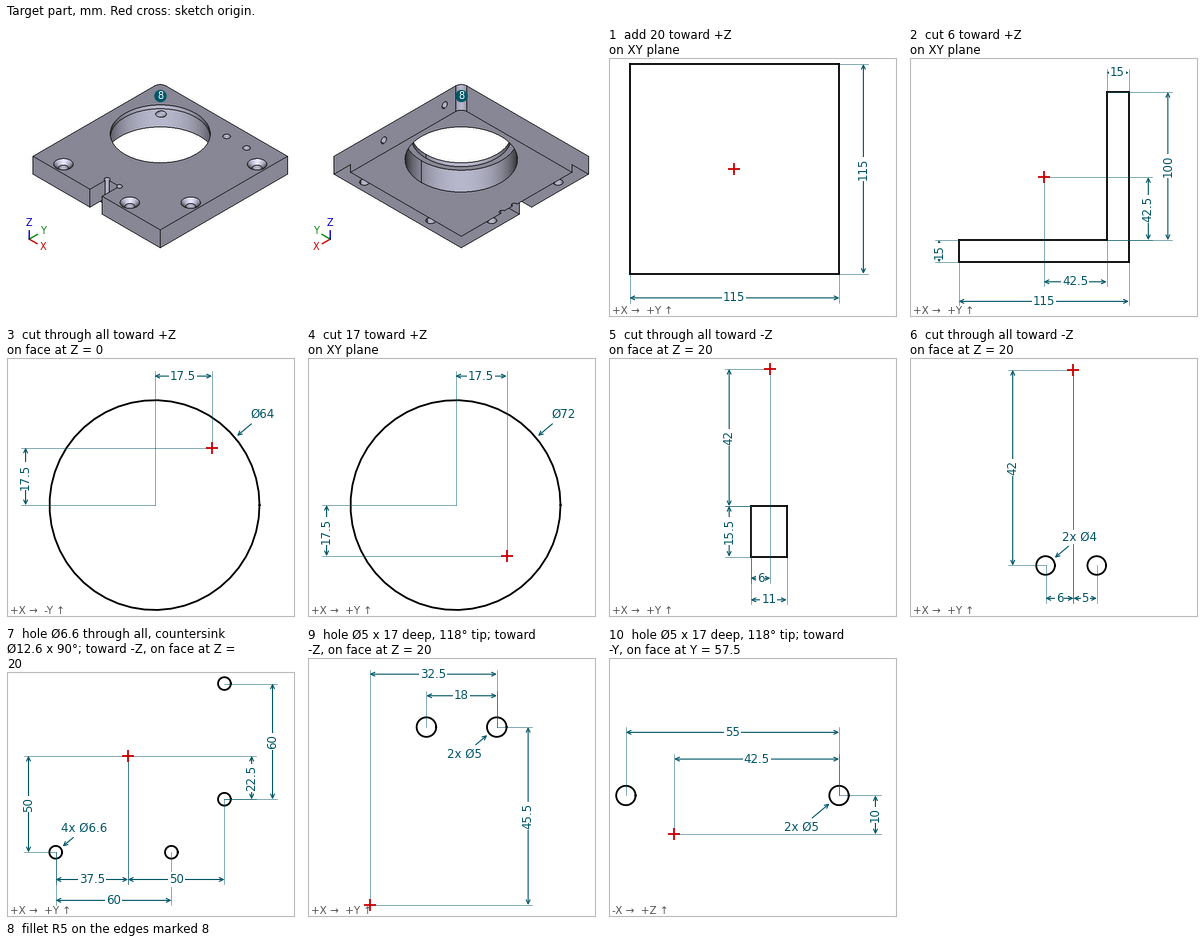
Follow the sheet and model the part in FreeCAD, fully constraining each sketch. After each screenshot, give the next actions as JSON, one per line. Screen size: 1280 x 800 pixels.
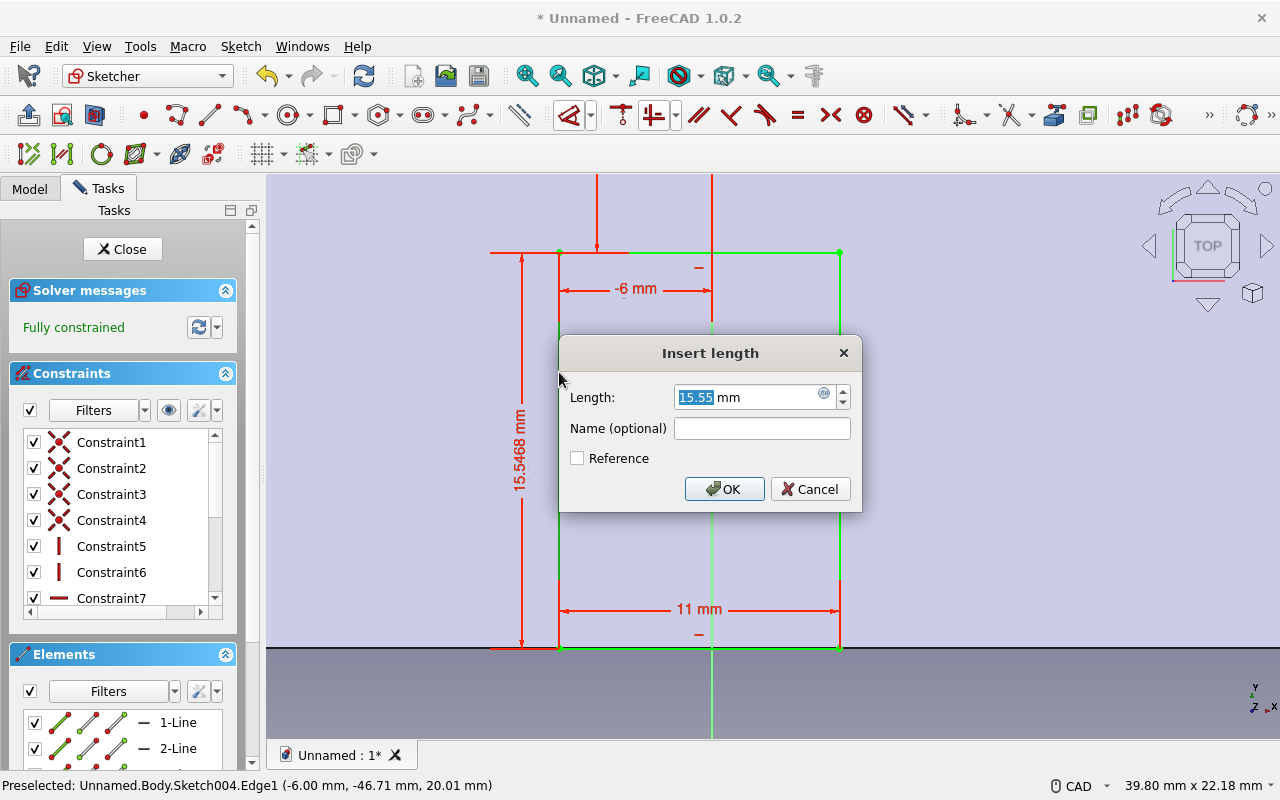
{"action": "type", "text": "15.5"}
{"action": "key", "text": "Return"}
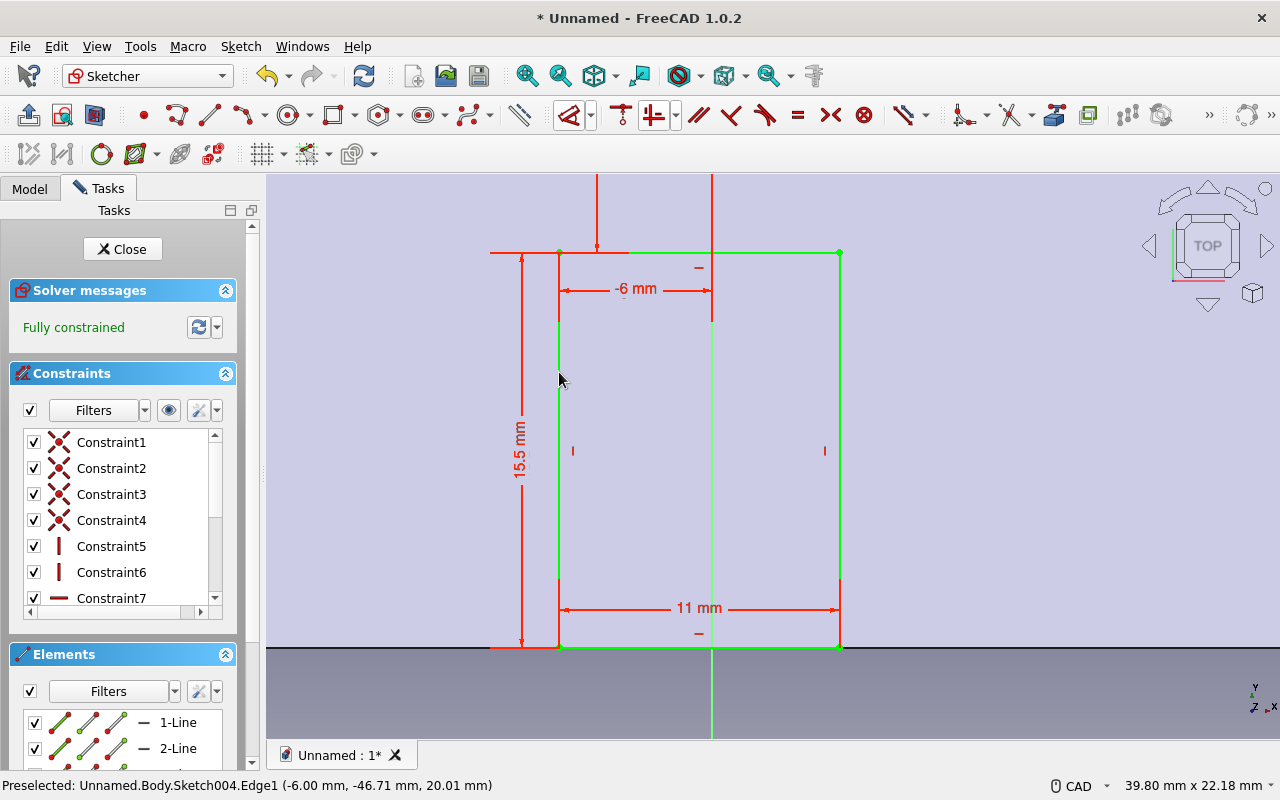
{"action": "left_click", "coordinate": [123, 249]}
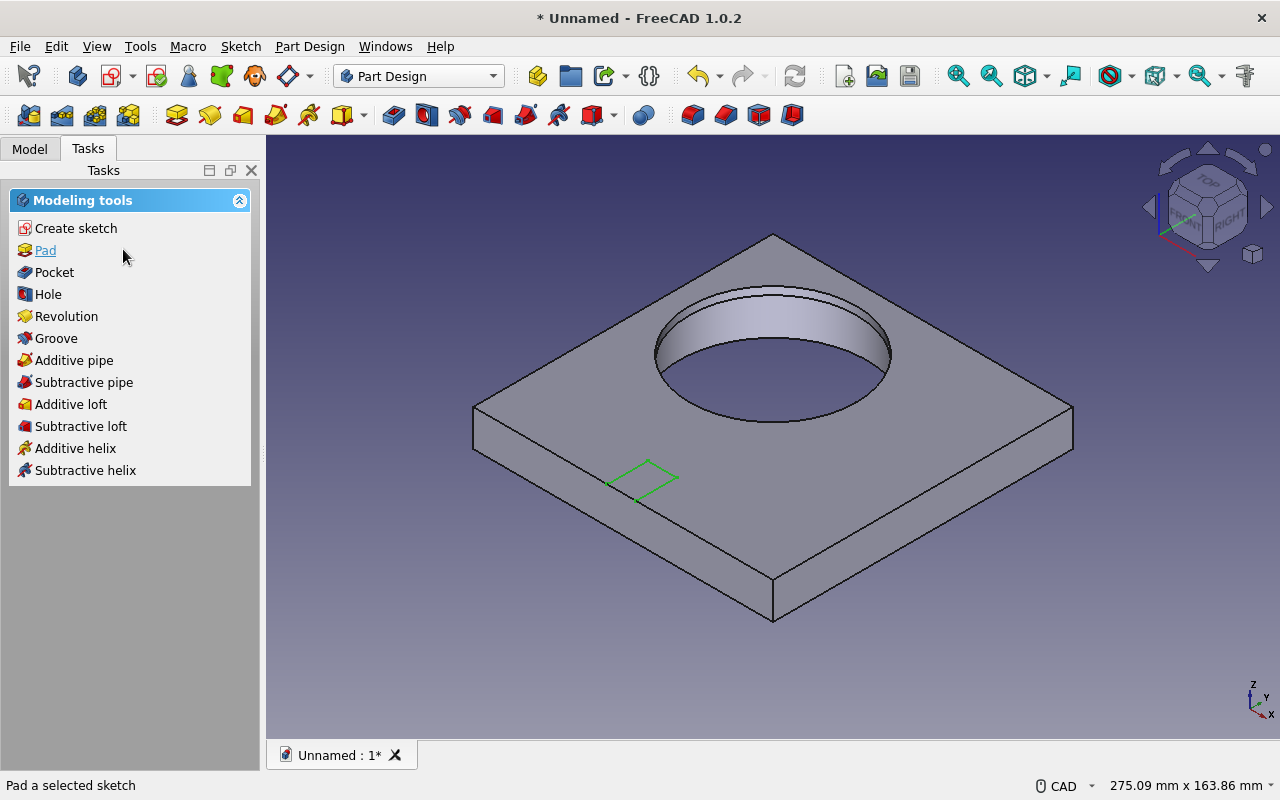
{"action": "left_click", "coordinate": [394, 116]}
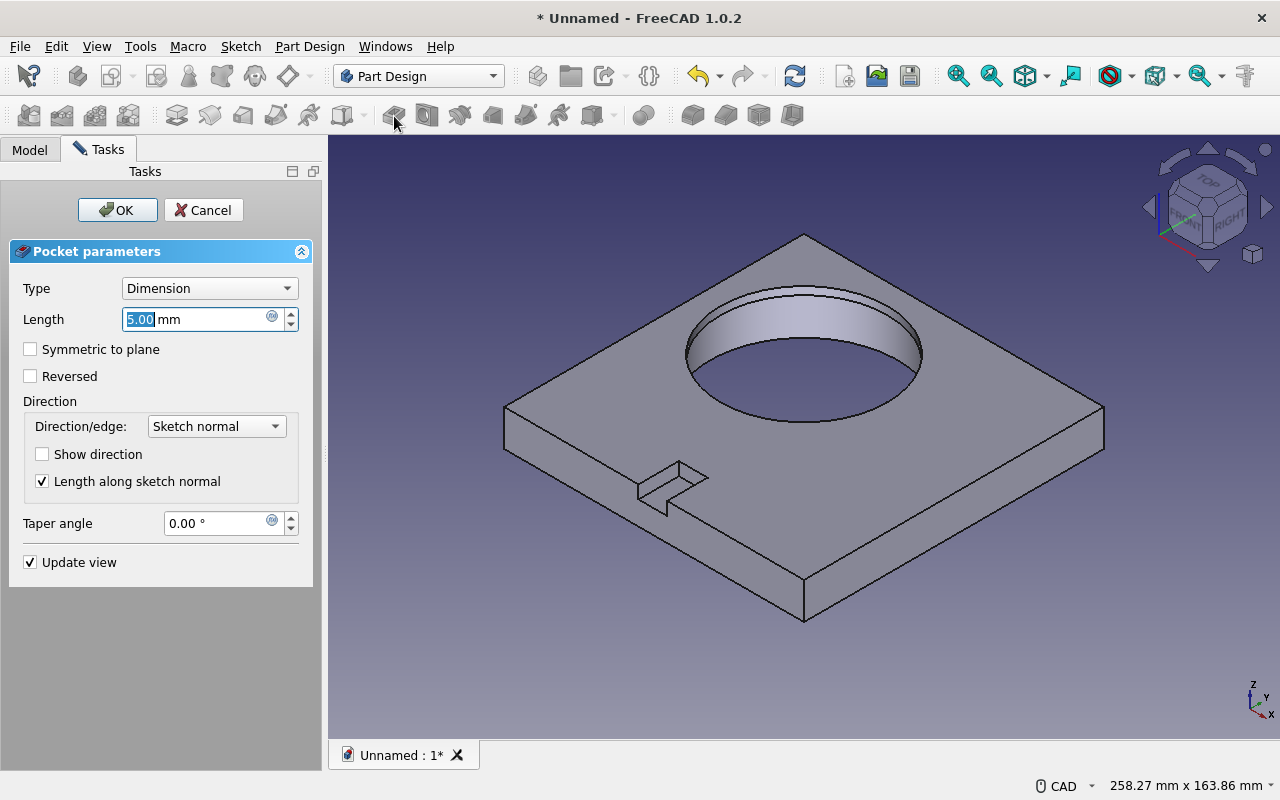
{"action": "left_click", "coordinate": [210, 288]}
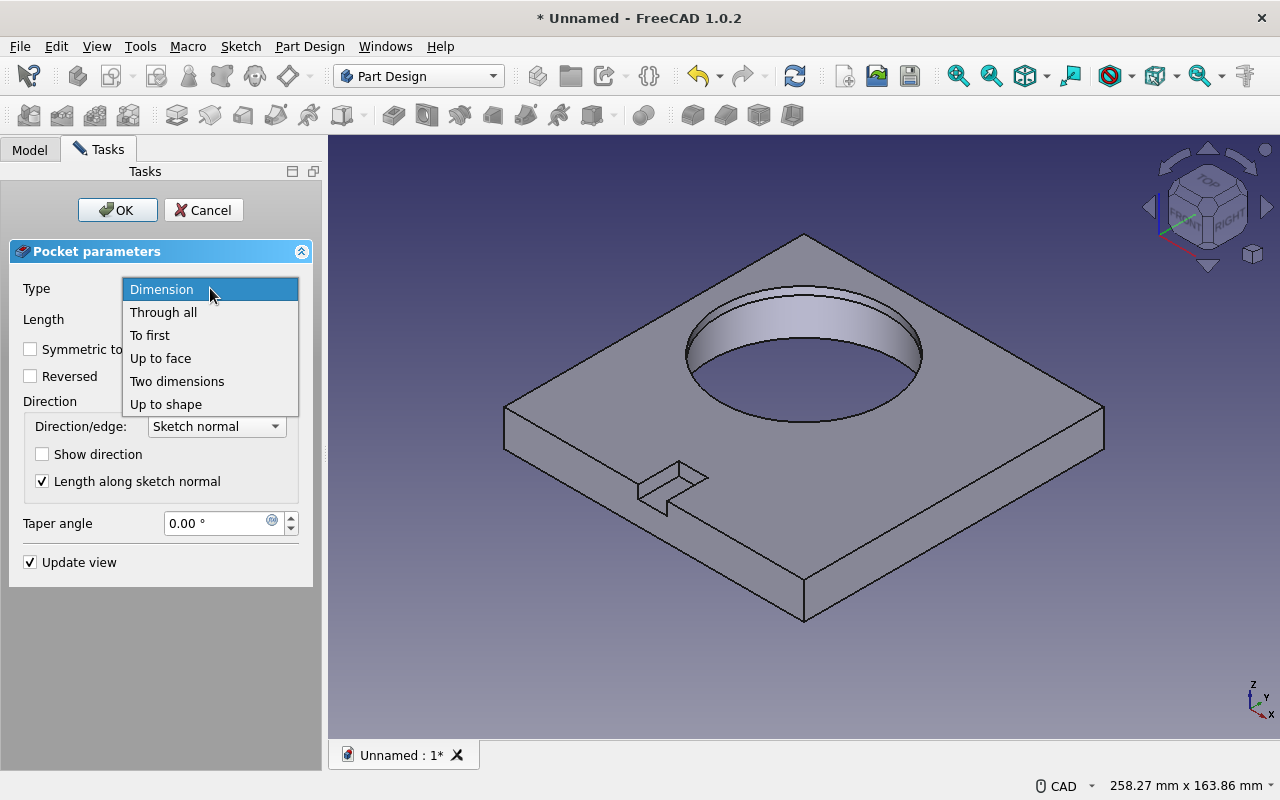
{"action": "left_click", "coordinate": [208, 312]}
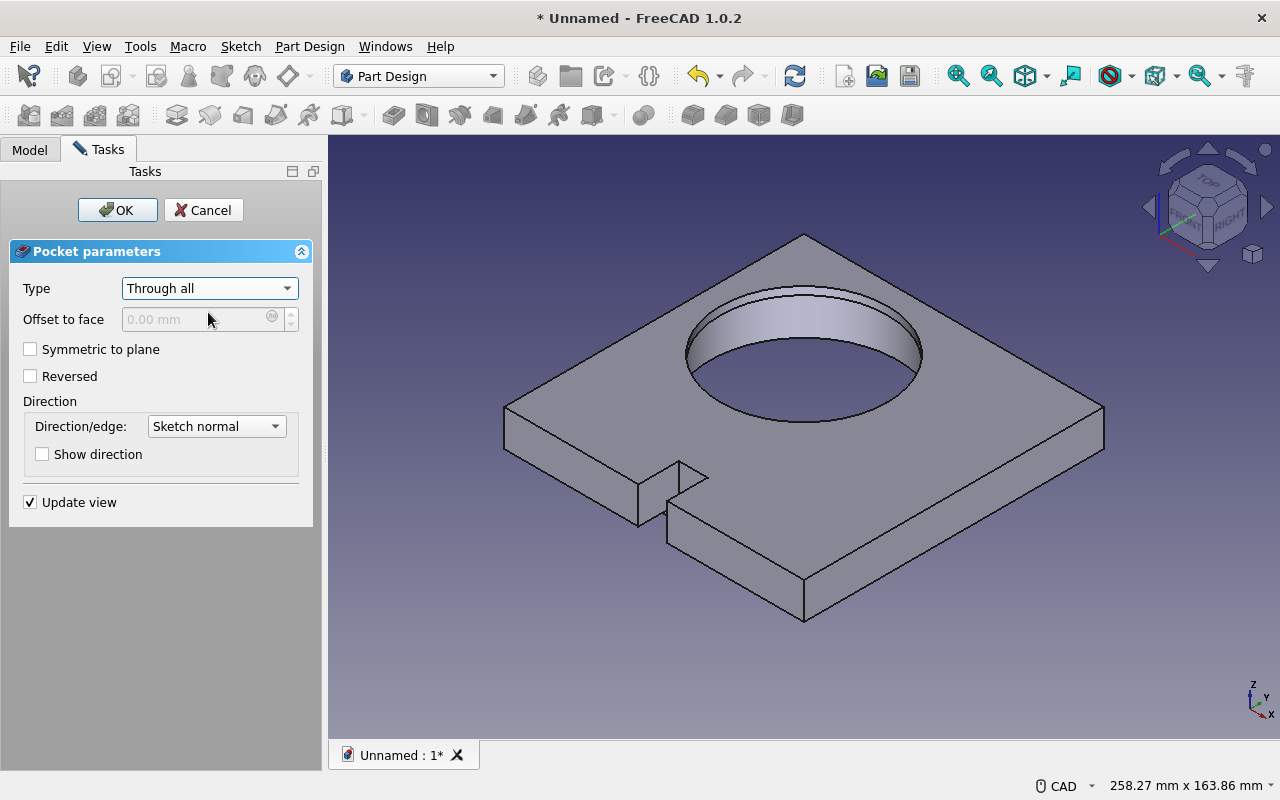
{"action": "left_click", "coordinate": [118, 210]}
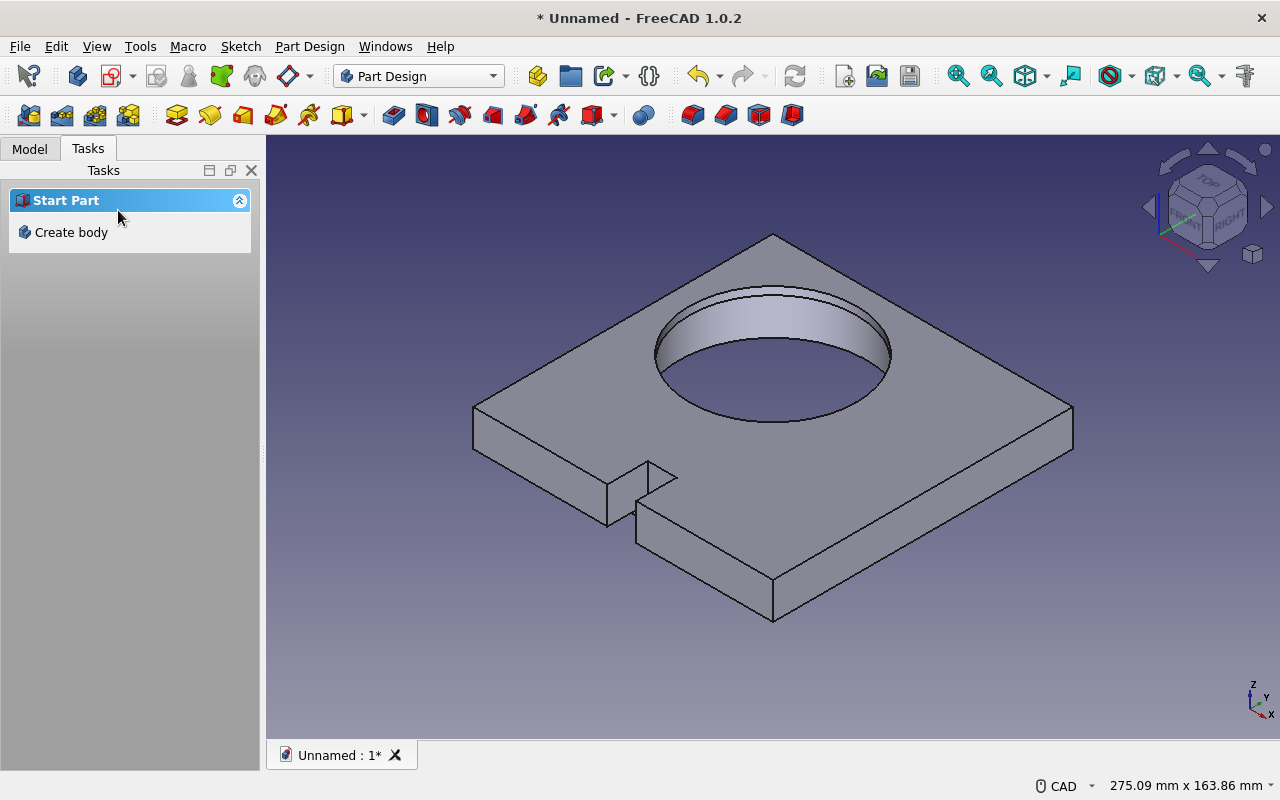
{"action": "left_click", "coordinate": [816, 480]}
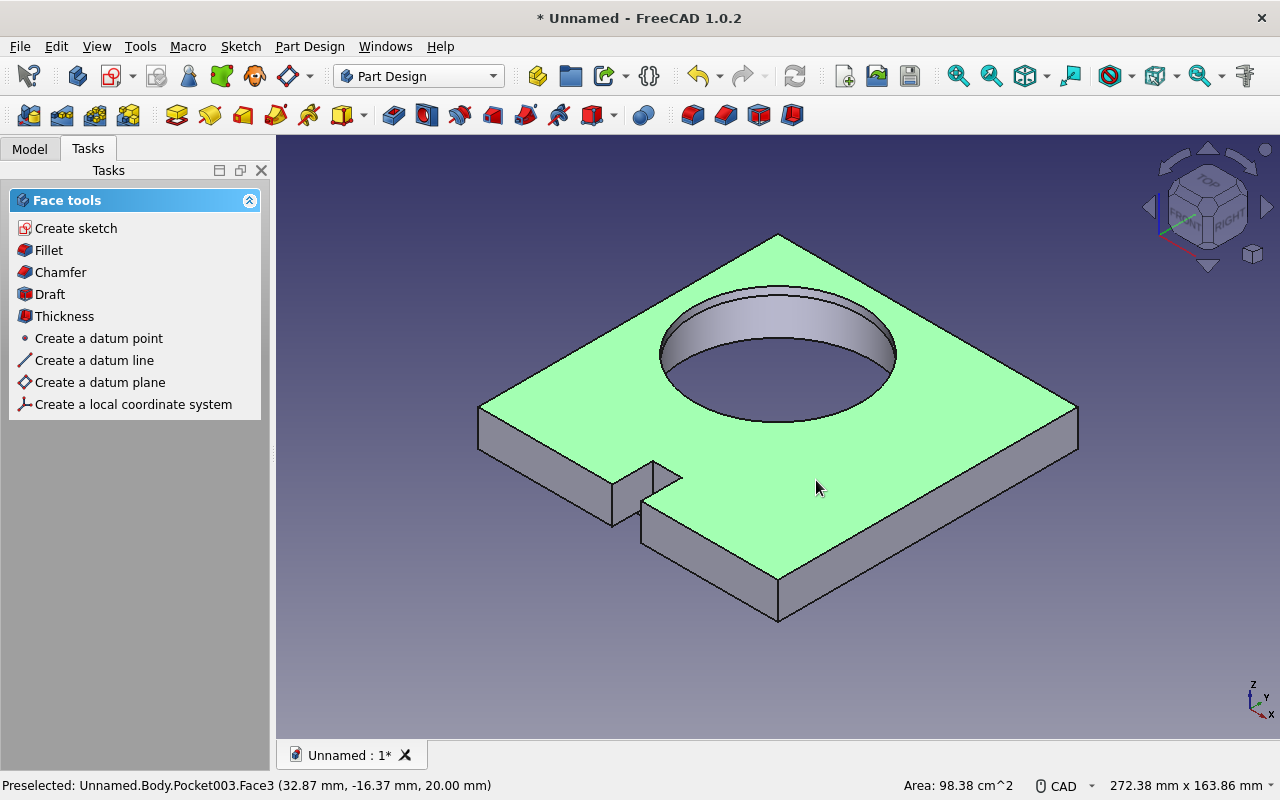
{"action": "left_click", "coordinate": [110, 76]}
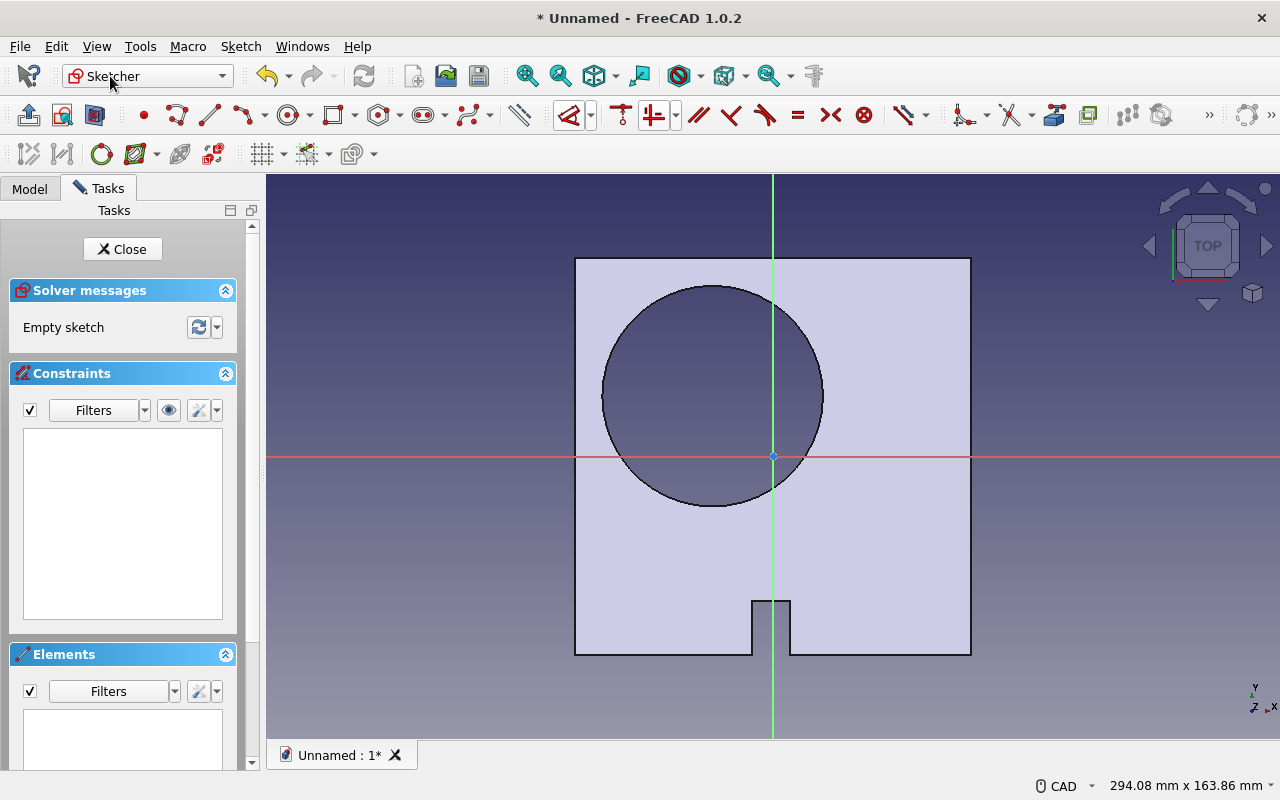
{"action": "scroll", "coordinate": [778, 616], "scroll_direction": "up", "scroll_amount": 12}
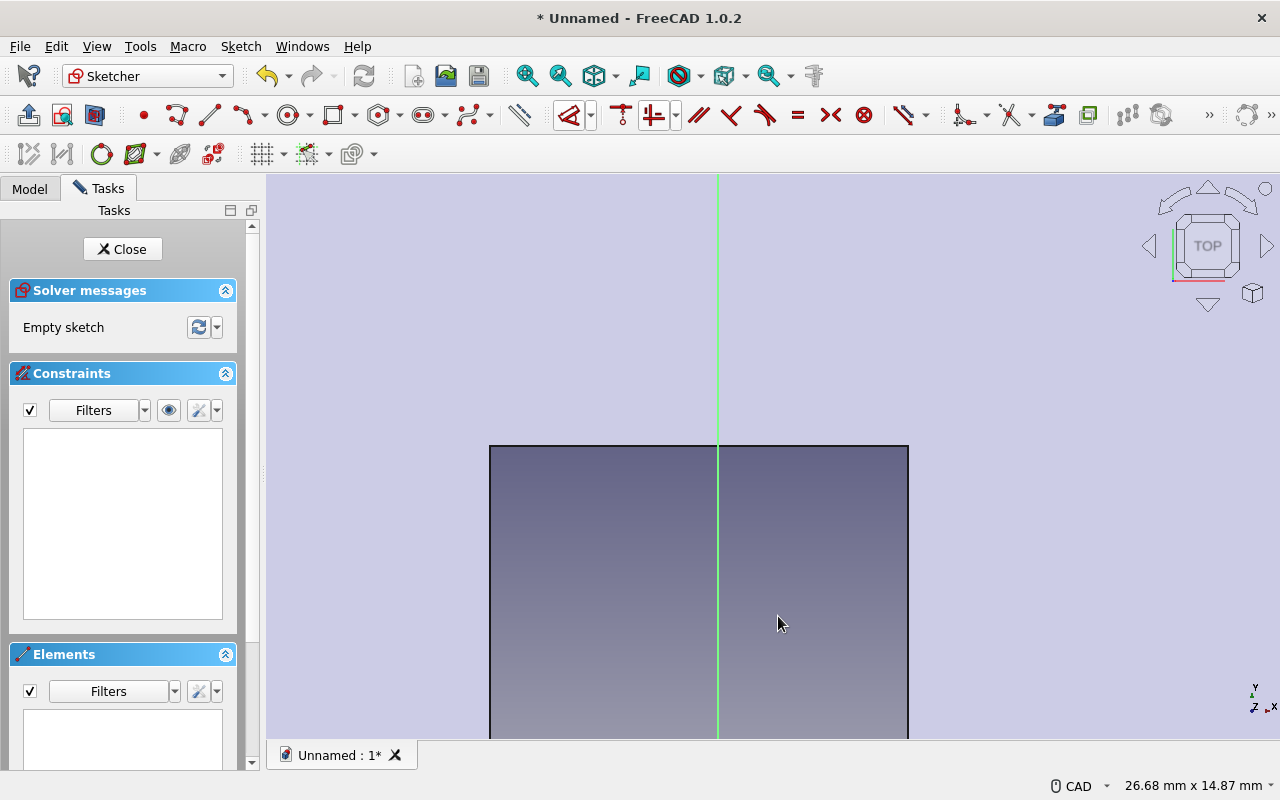
{"action": "left_click", "coordinate": [288, 116]}